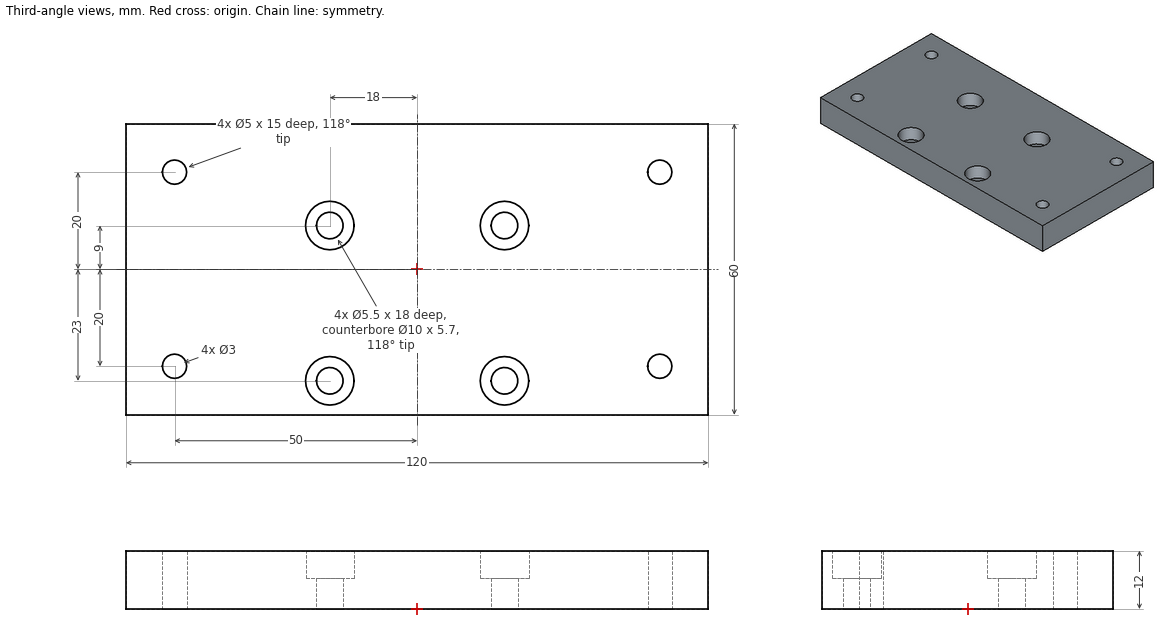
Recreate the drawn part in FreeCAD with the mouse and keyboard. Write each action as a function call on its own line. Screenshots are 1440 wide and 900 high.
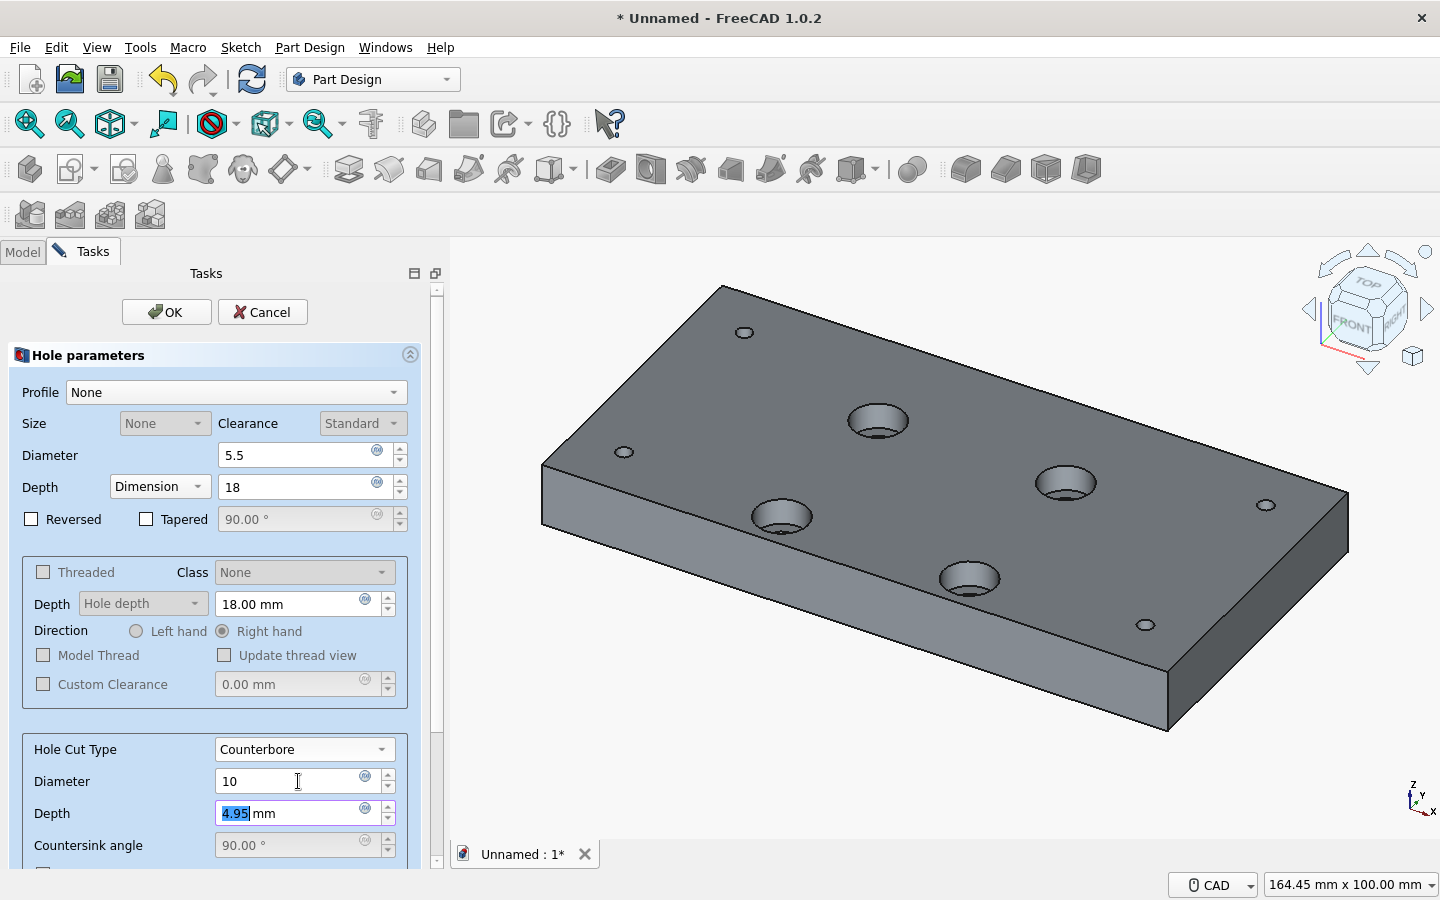
text(5.7)
key(Tab)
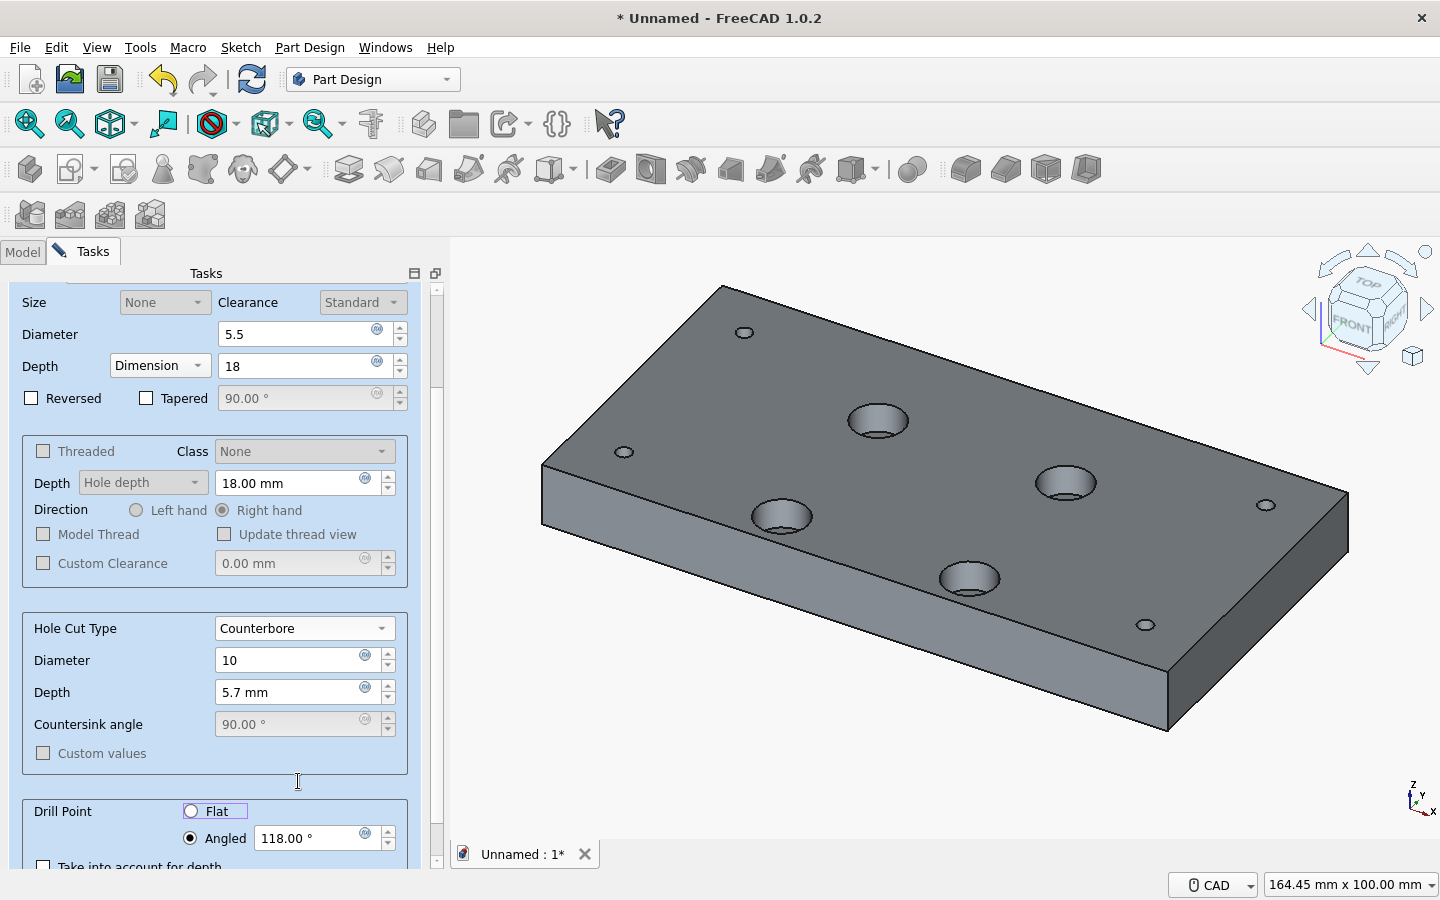
scroll(437, 576, up, 3)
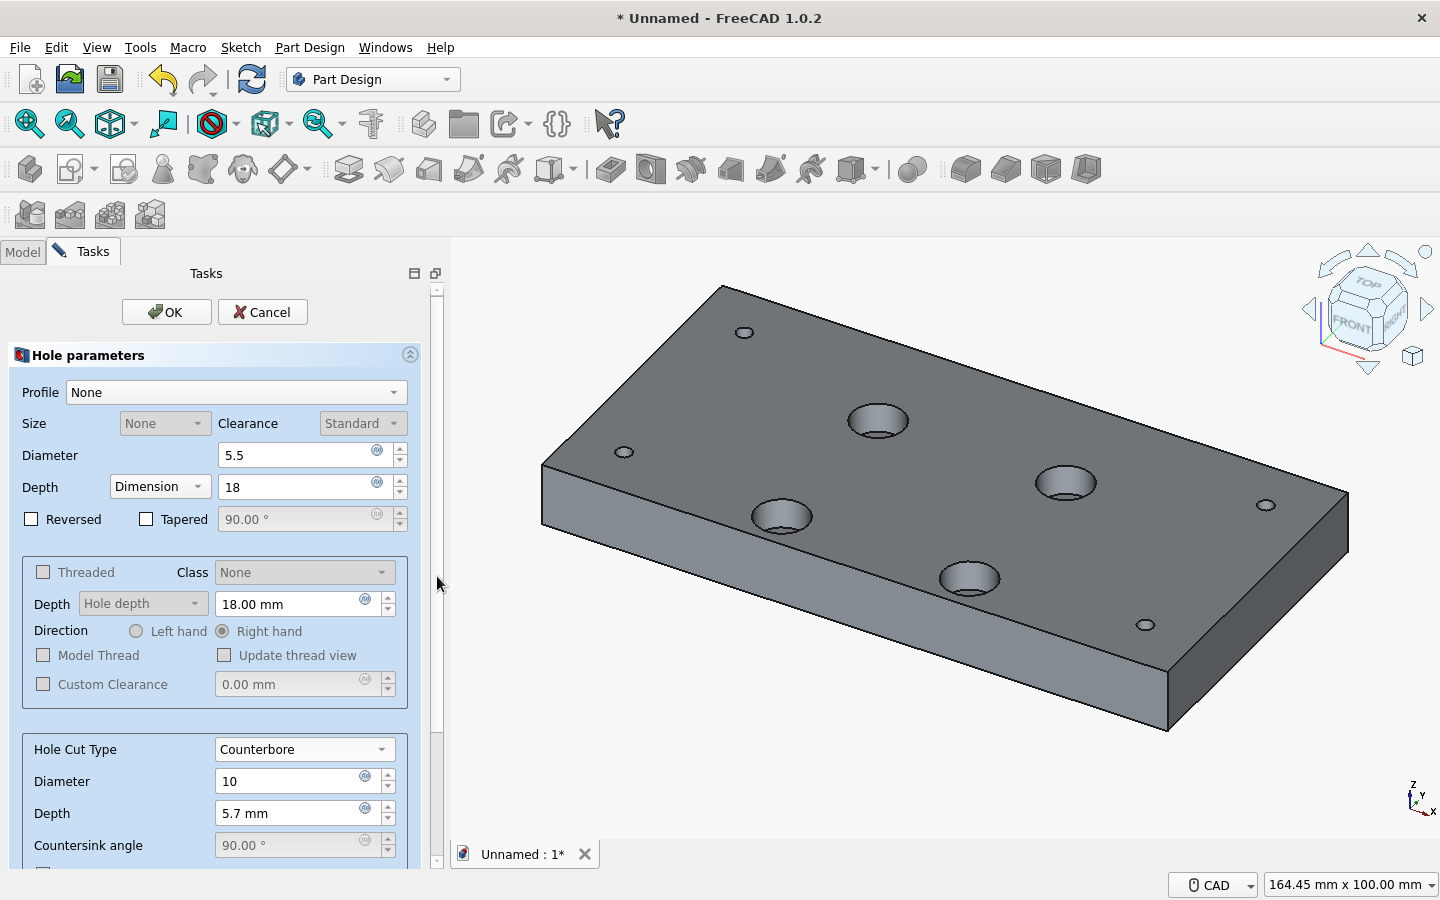
click(167, 312)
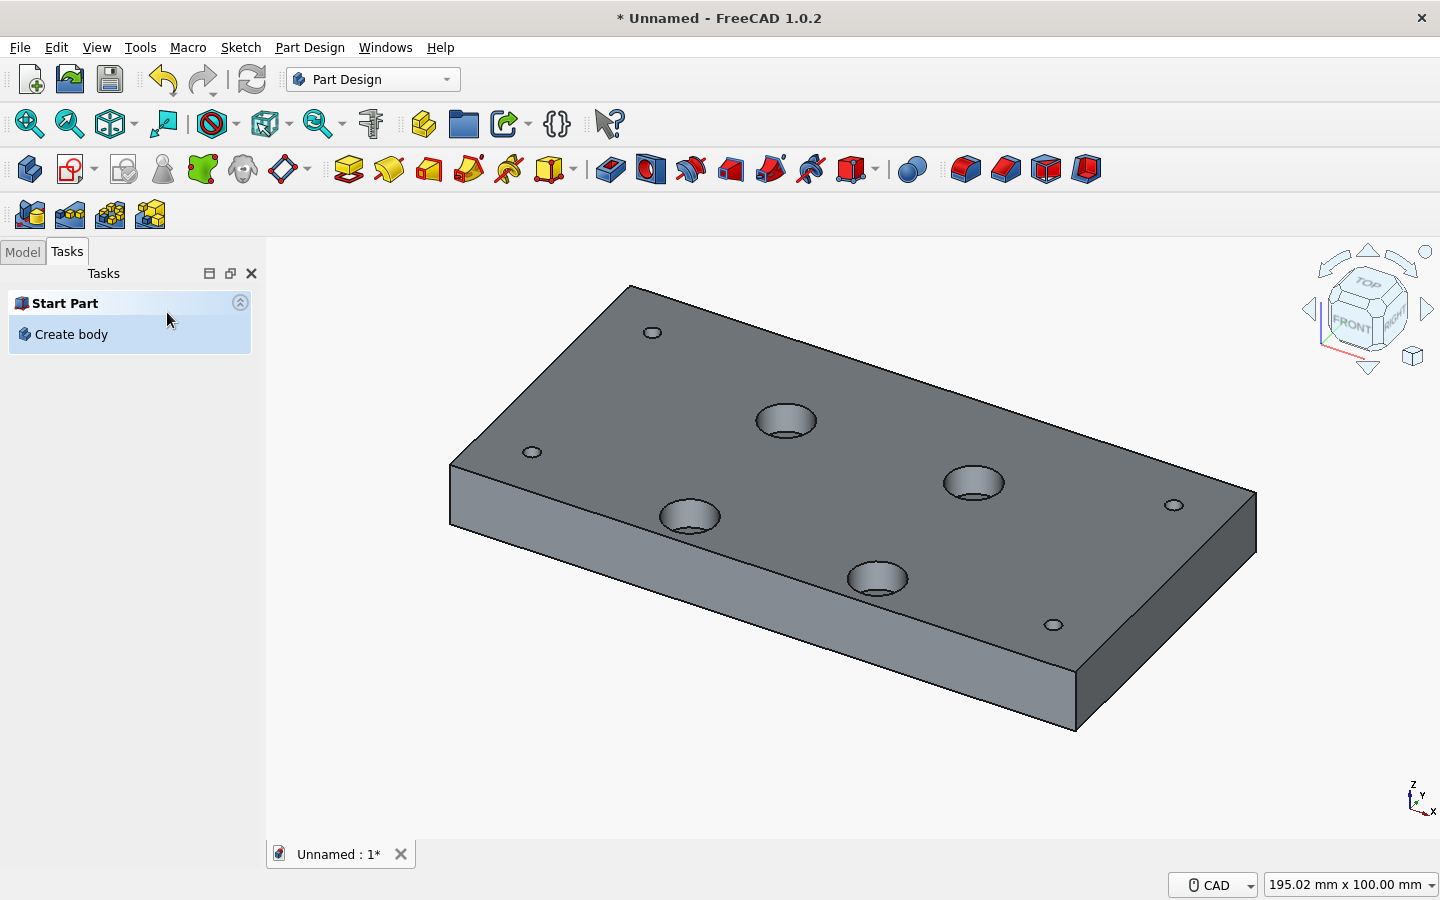
click(827, 503)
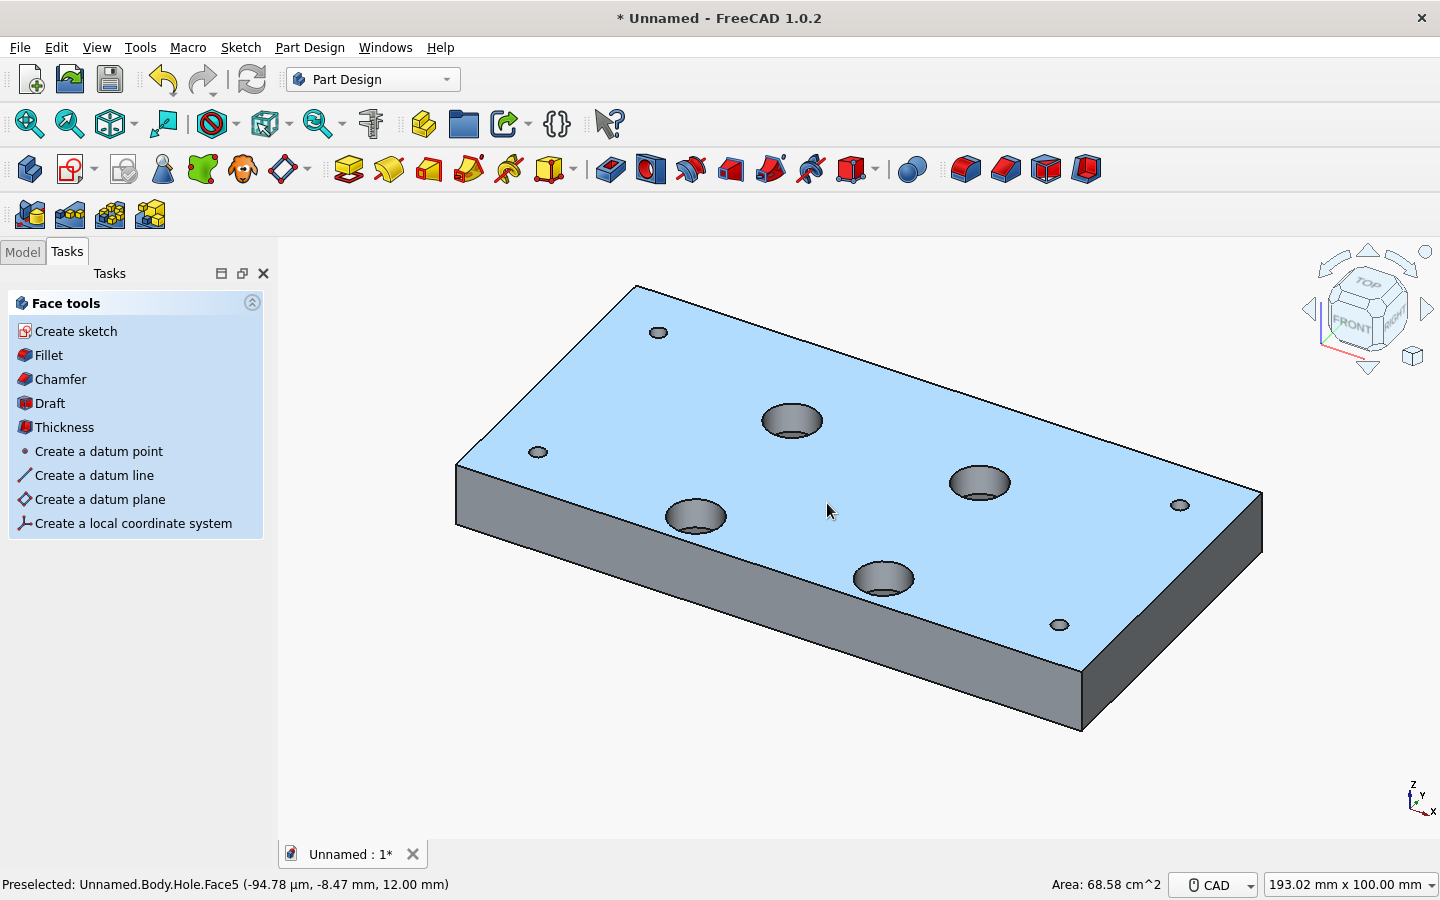
click(70, 170)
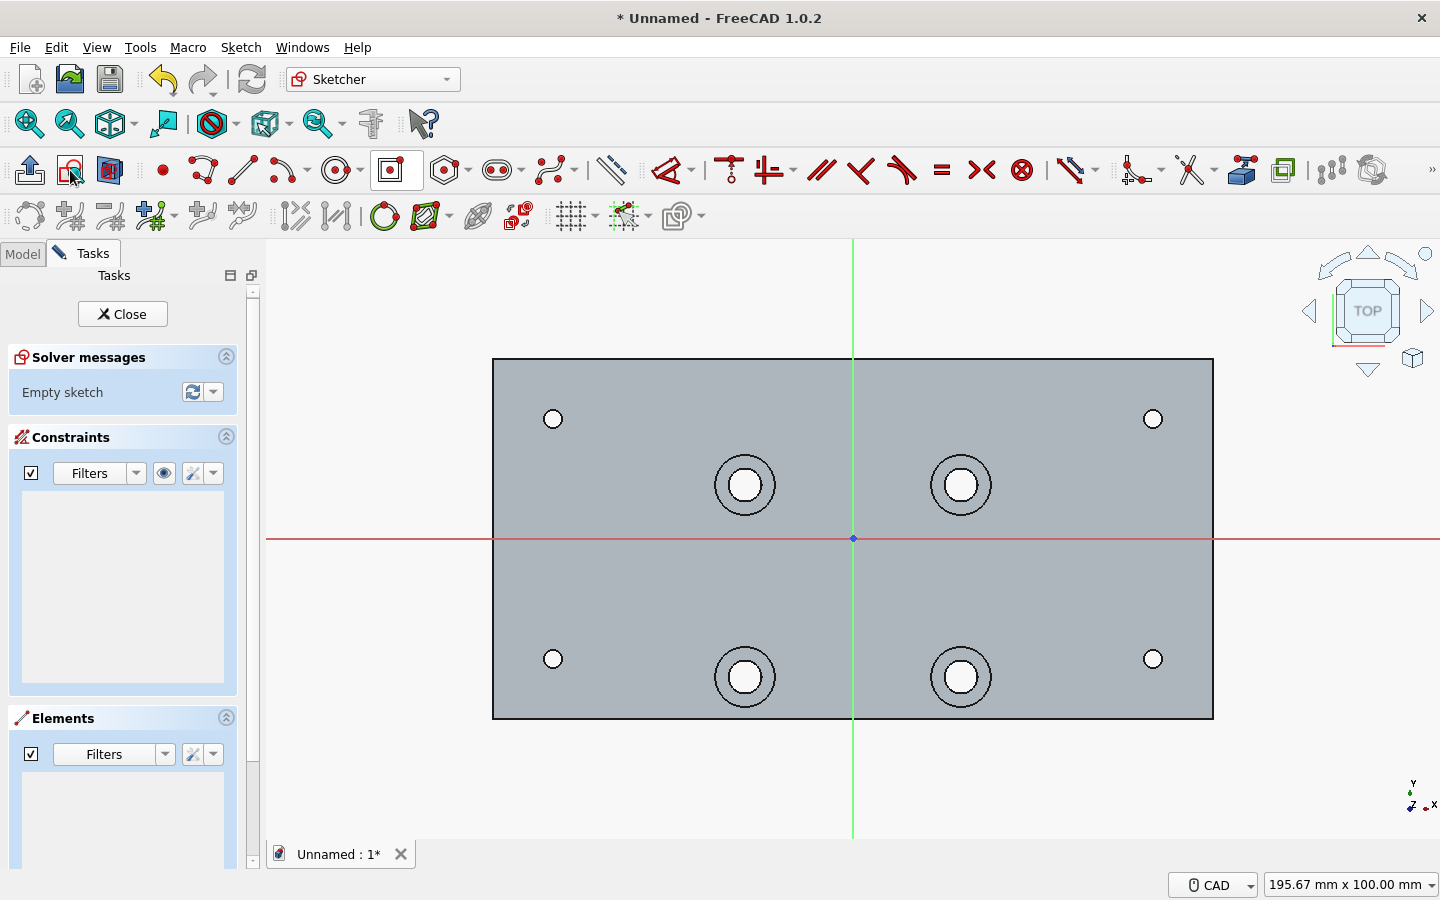
click(336, 170)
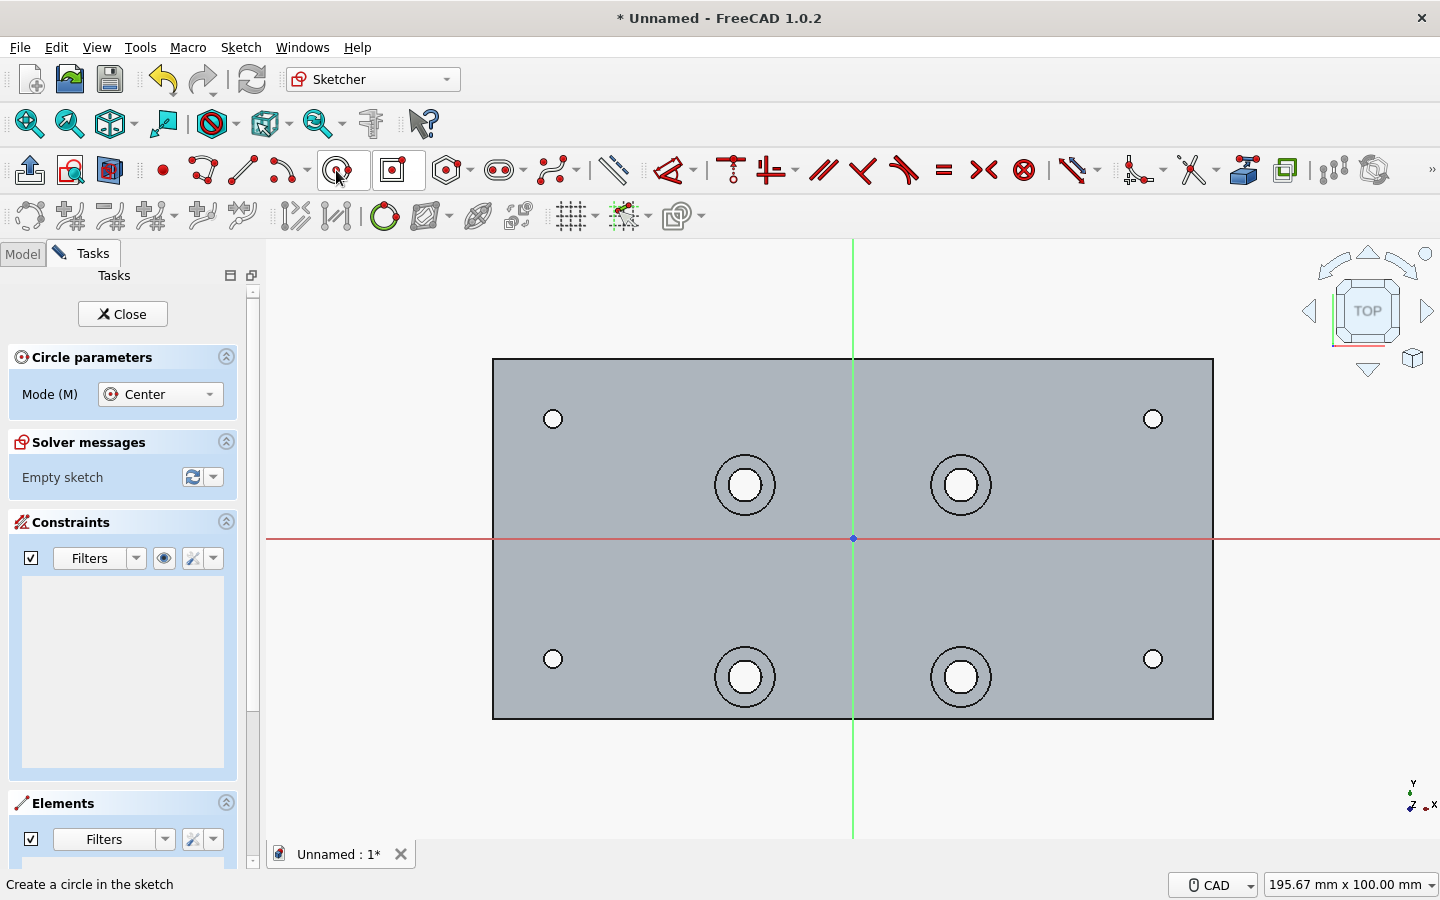
scroll(553, 419, up, 3)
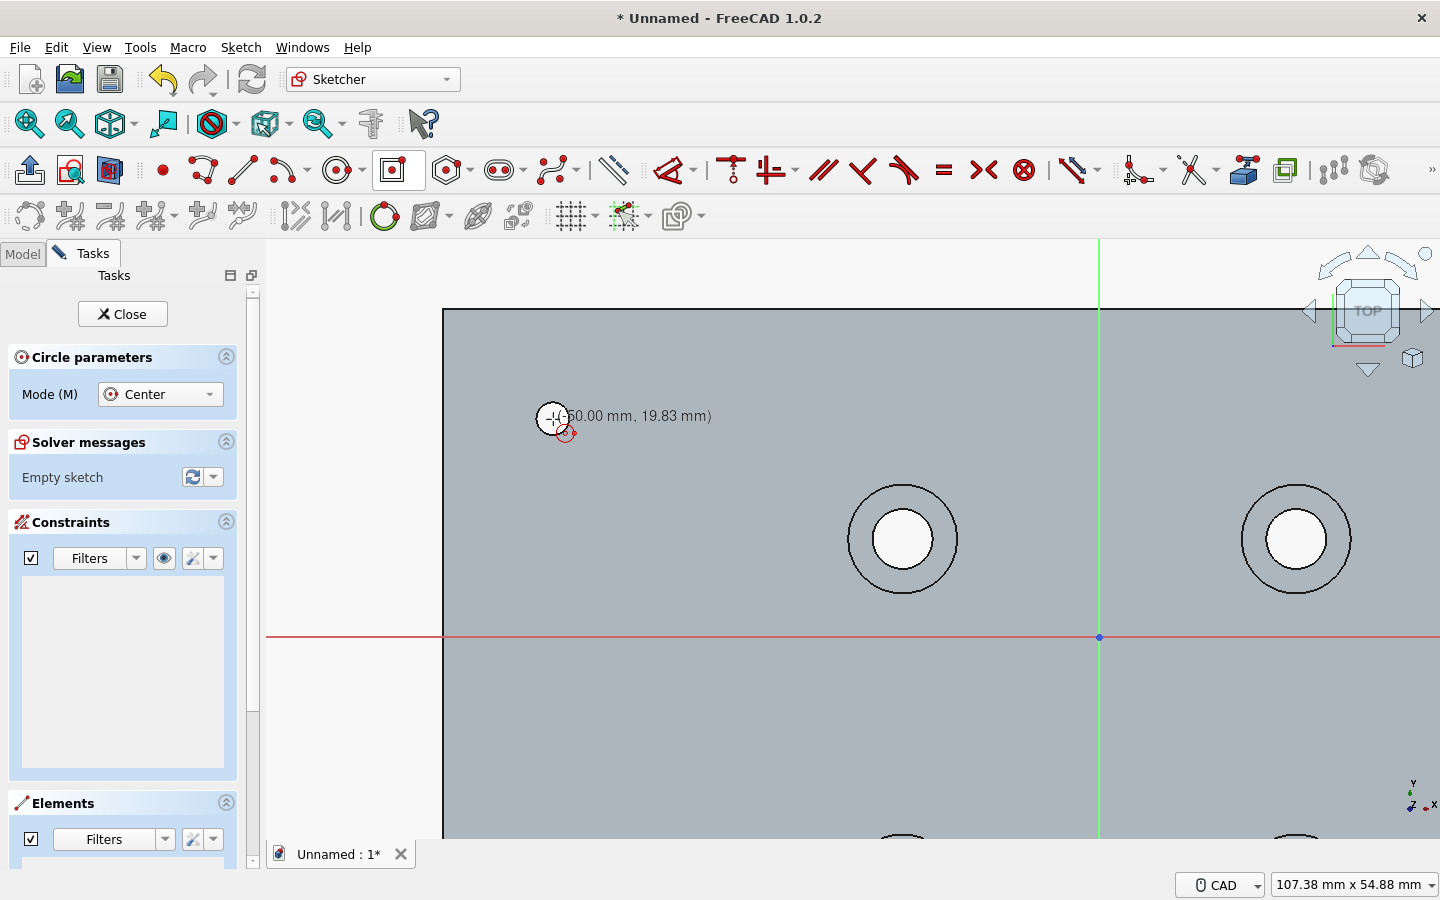
click(553, 419)
click(572, 399)